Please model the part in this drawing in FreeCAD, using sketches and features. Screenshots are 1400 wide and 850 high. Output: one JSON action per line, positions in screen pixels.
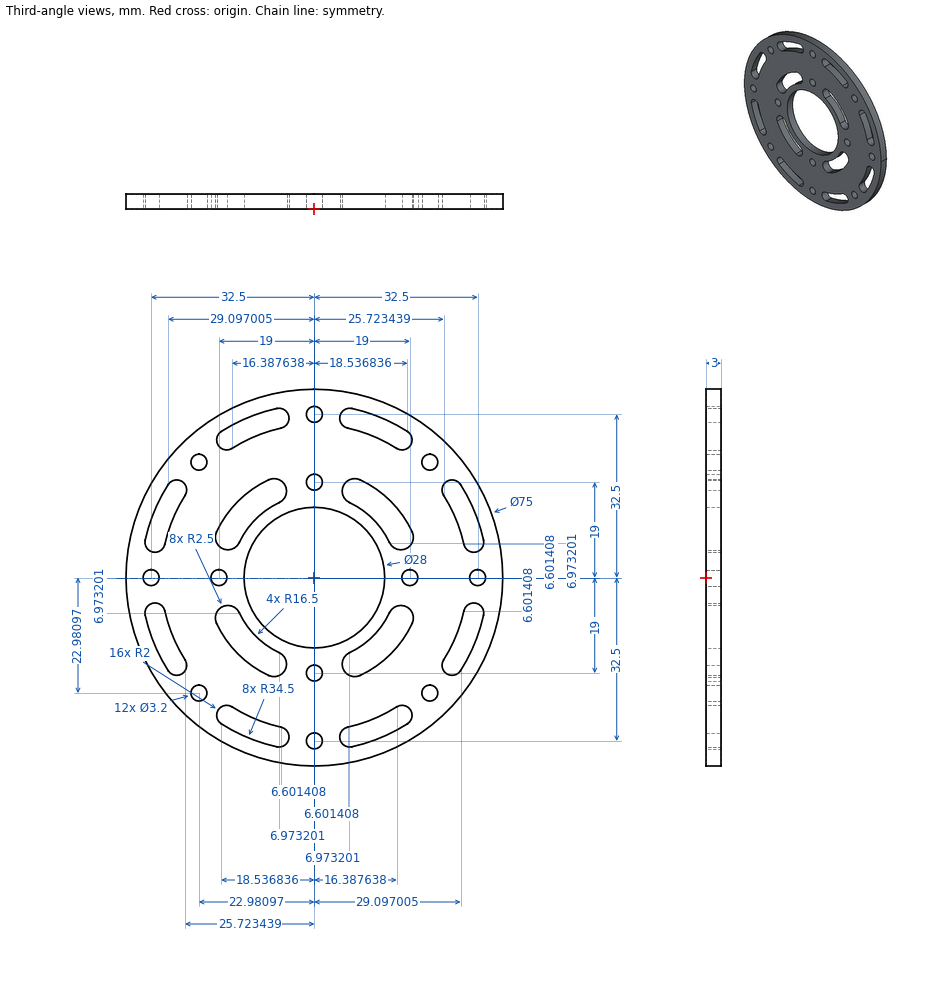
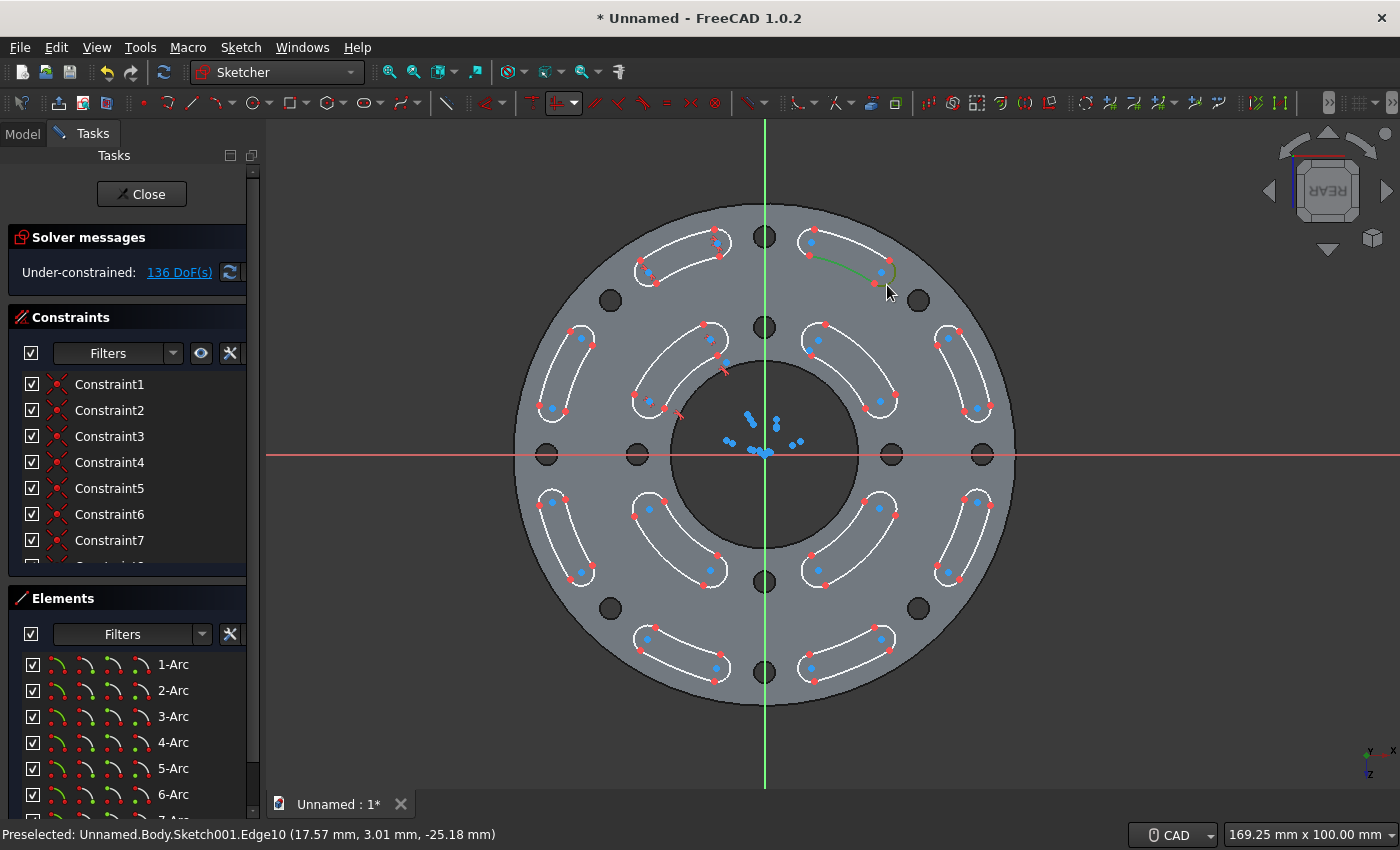
{"action": "left_click", "coordinate": [644, 104]}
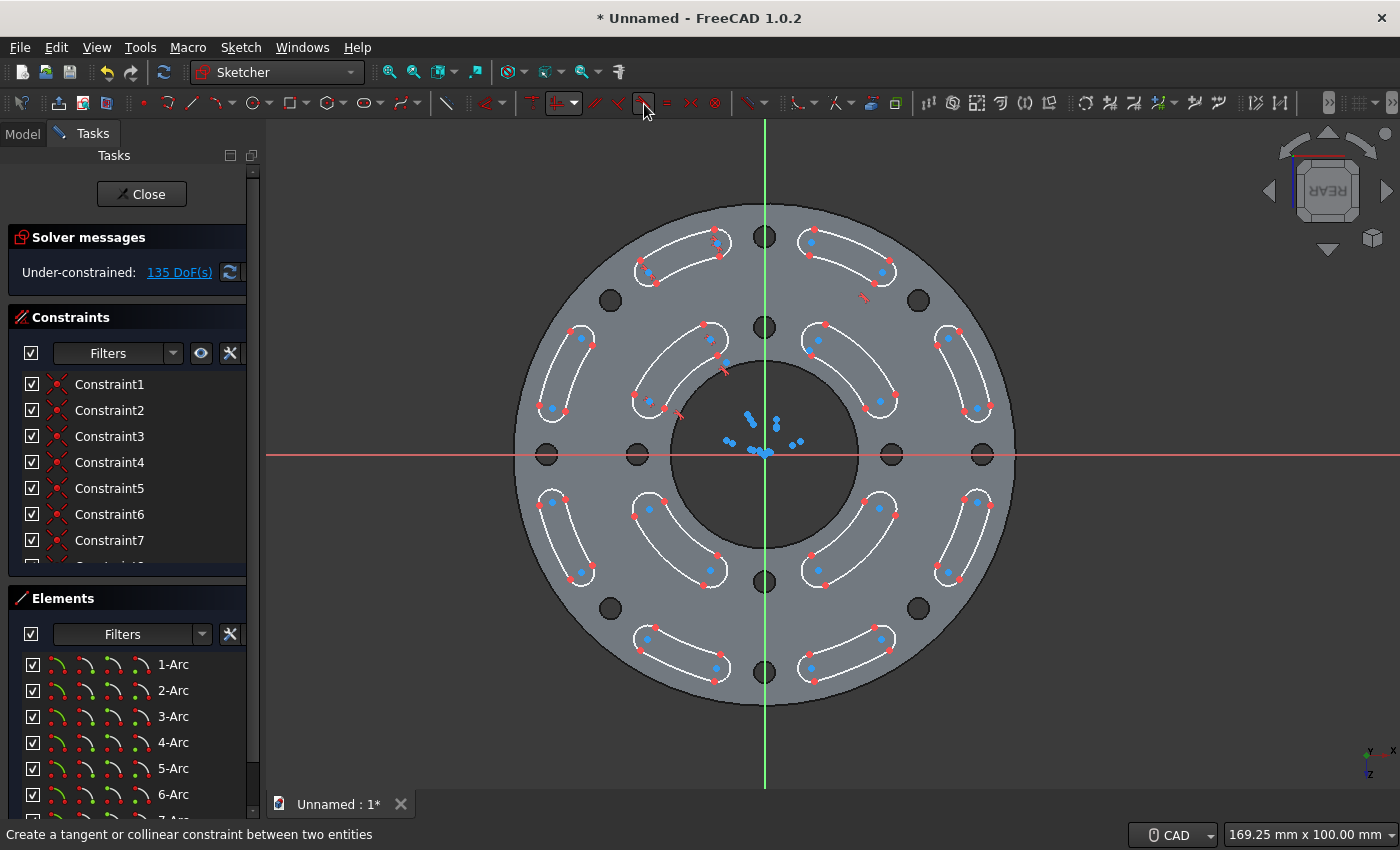
{"action": "left_click", "coordinate": [856, 272]}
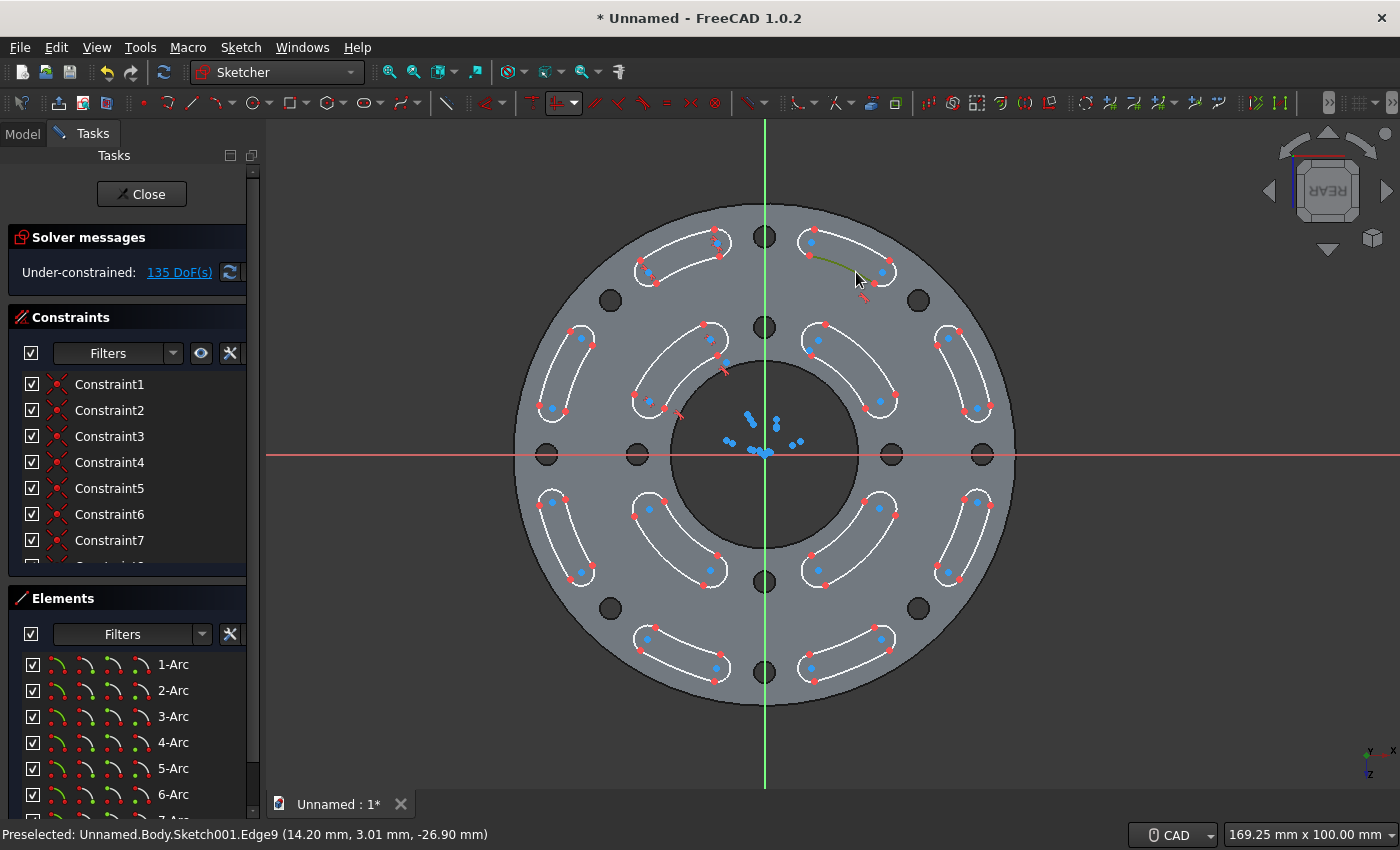
{"action": "left_click", "coordinate": [802, 233]}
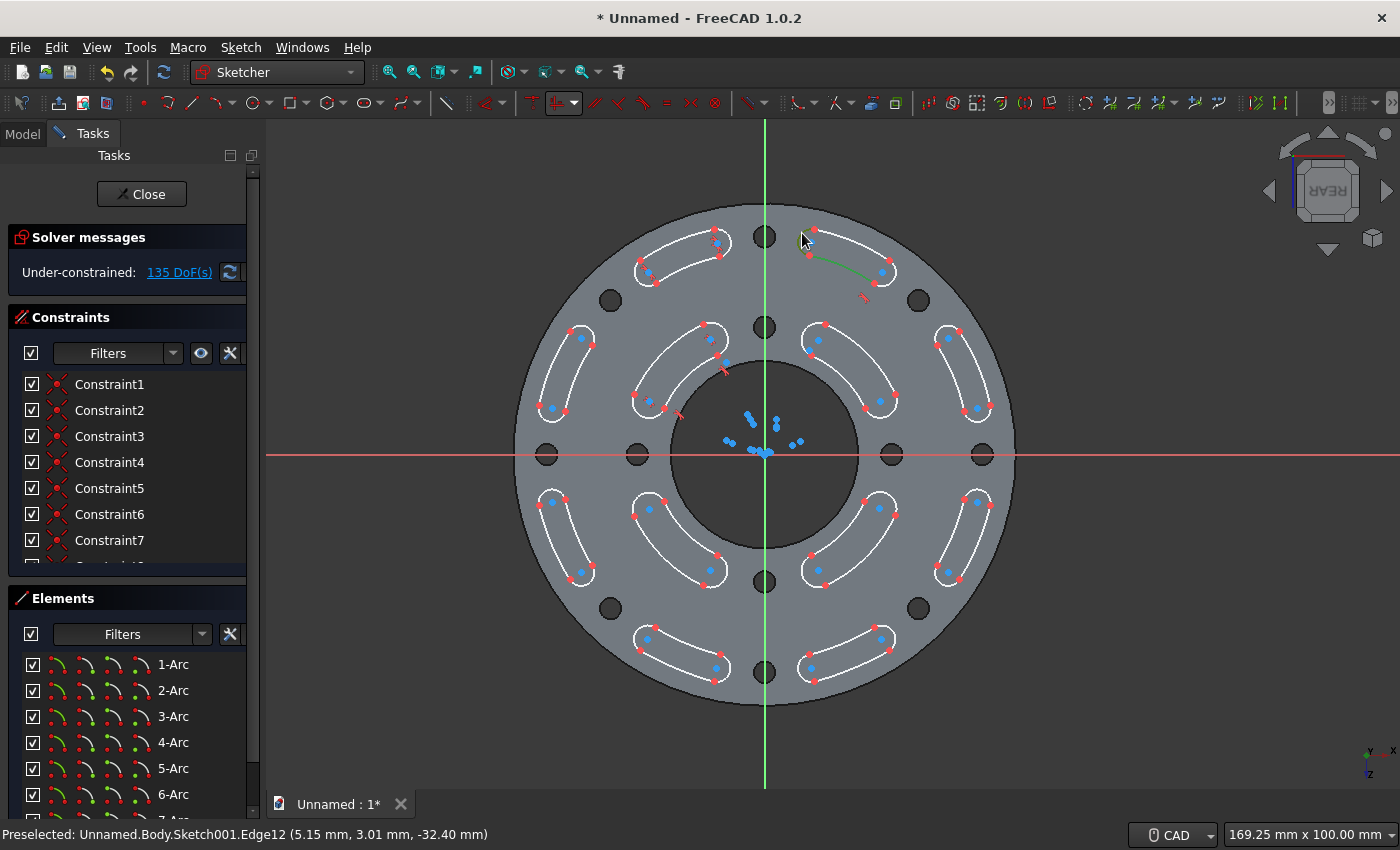
{"action": "left_click", "coordinate": [644, 104]}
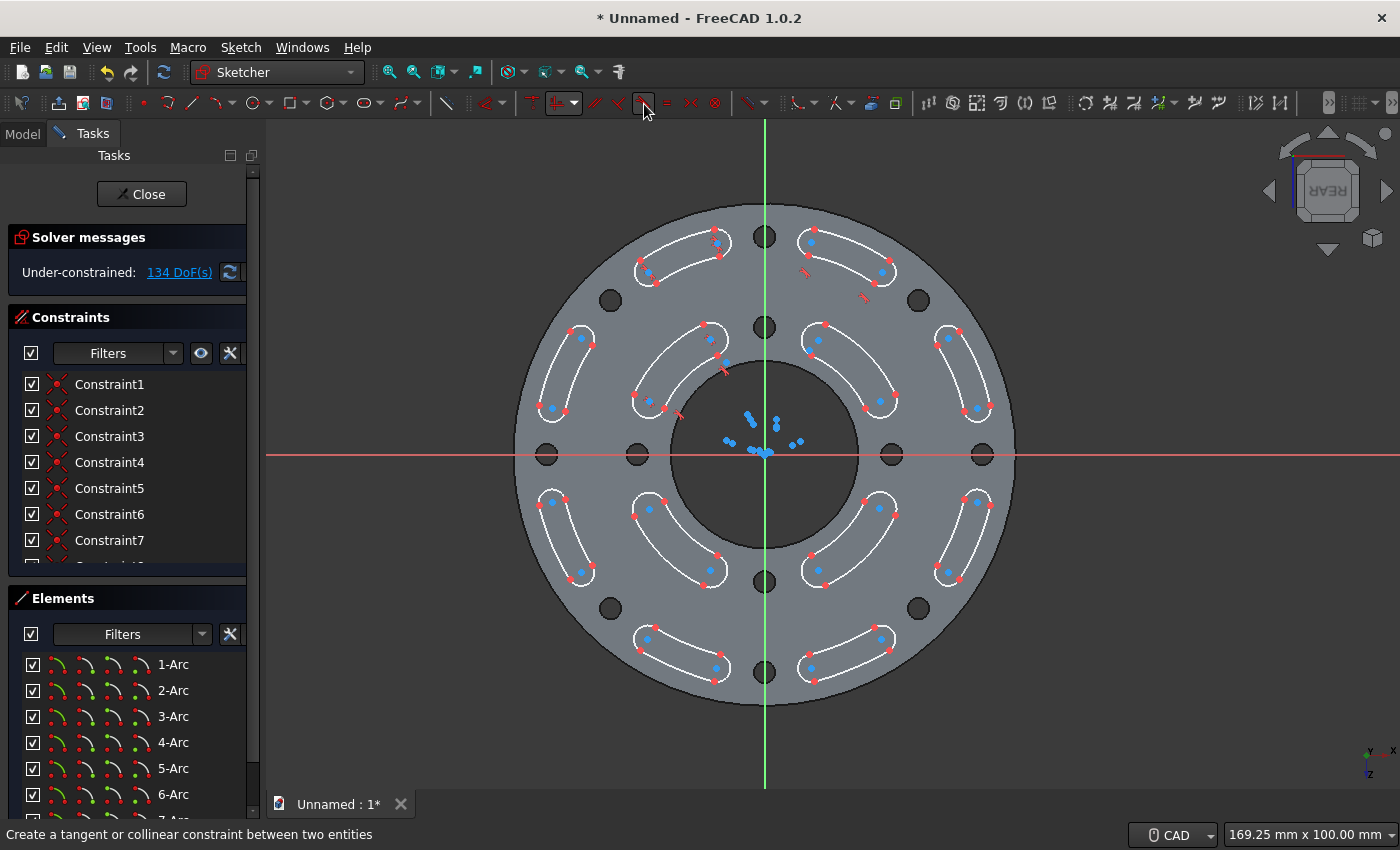
{"action": "left_click", "coordinate": [887, 285]}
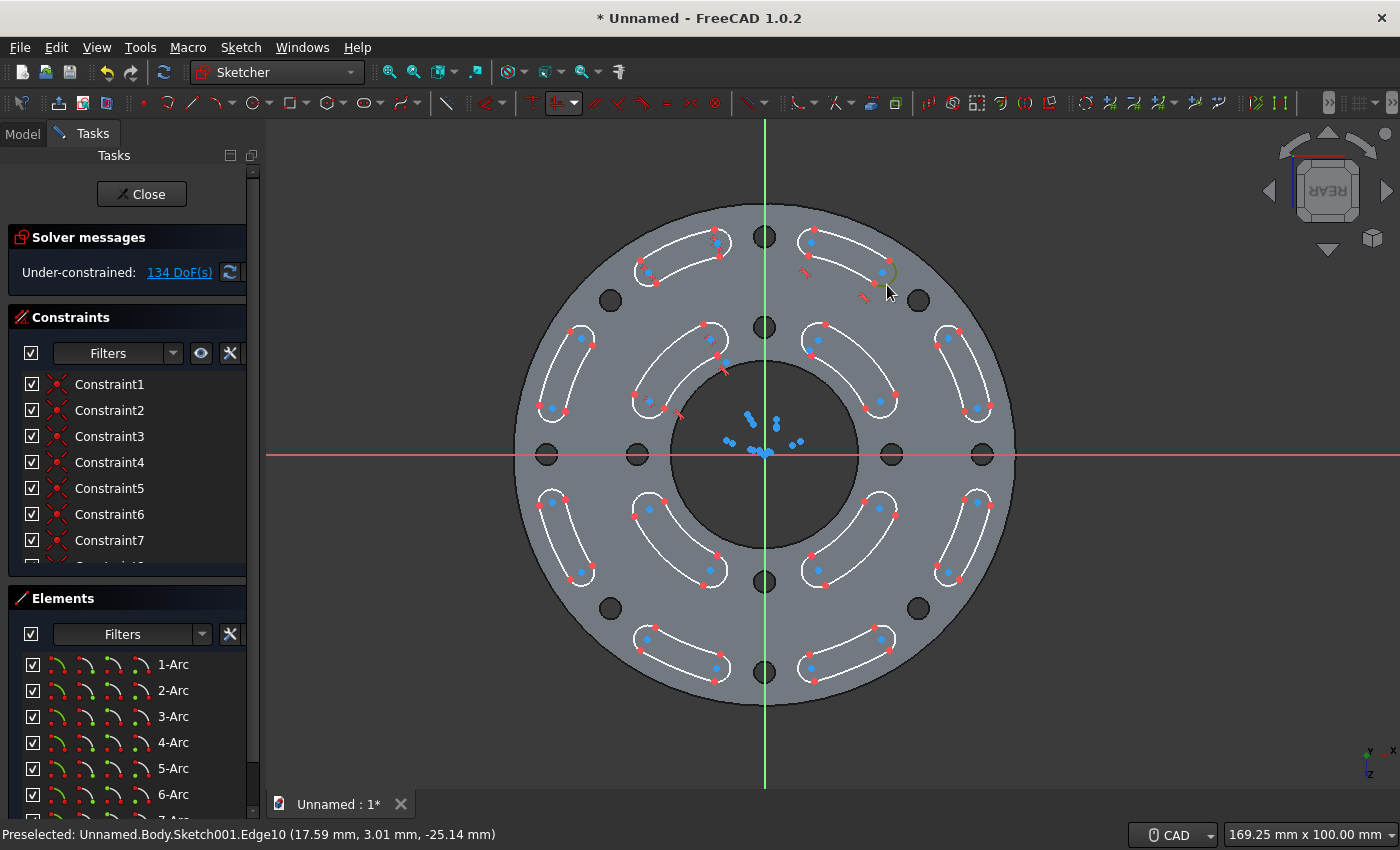
{"action": "left_click", "coordinate": [868, 248]}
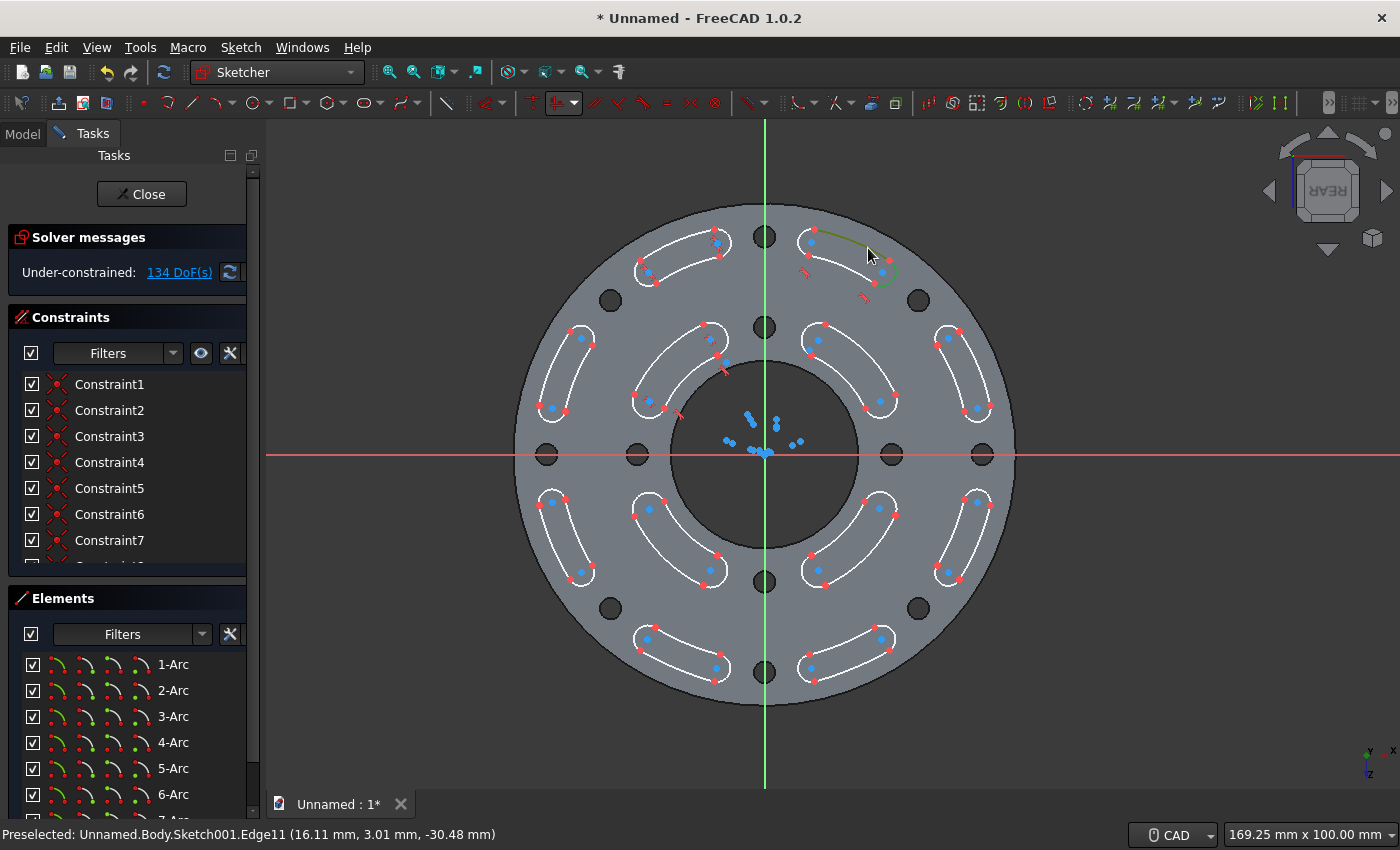
{"action": "left_click", "coordinate": [644, 104]}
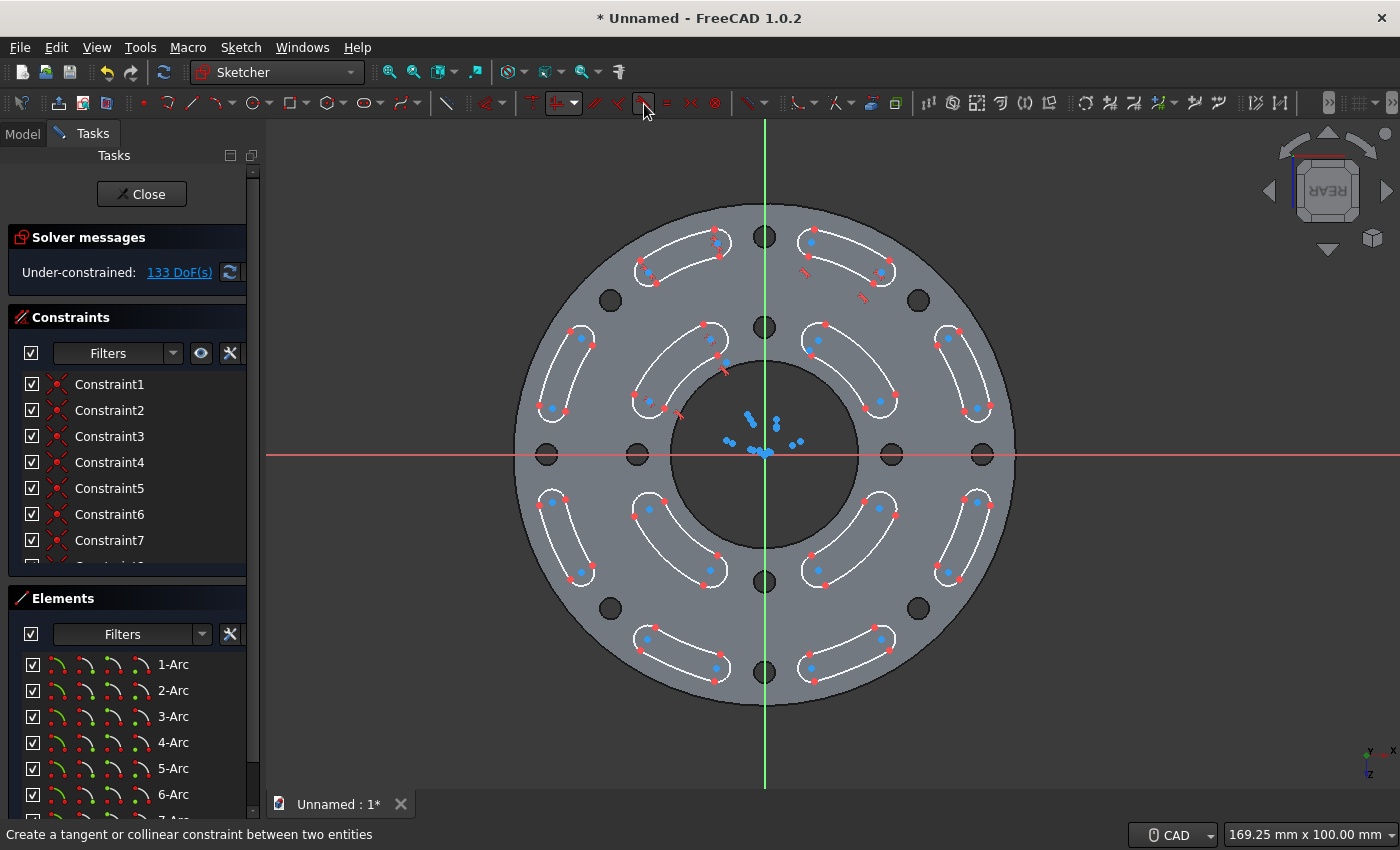
{"action": "left_click", "coordinate": [868, 248]}